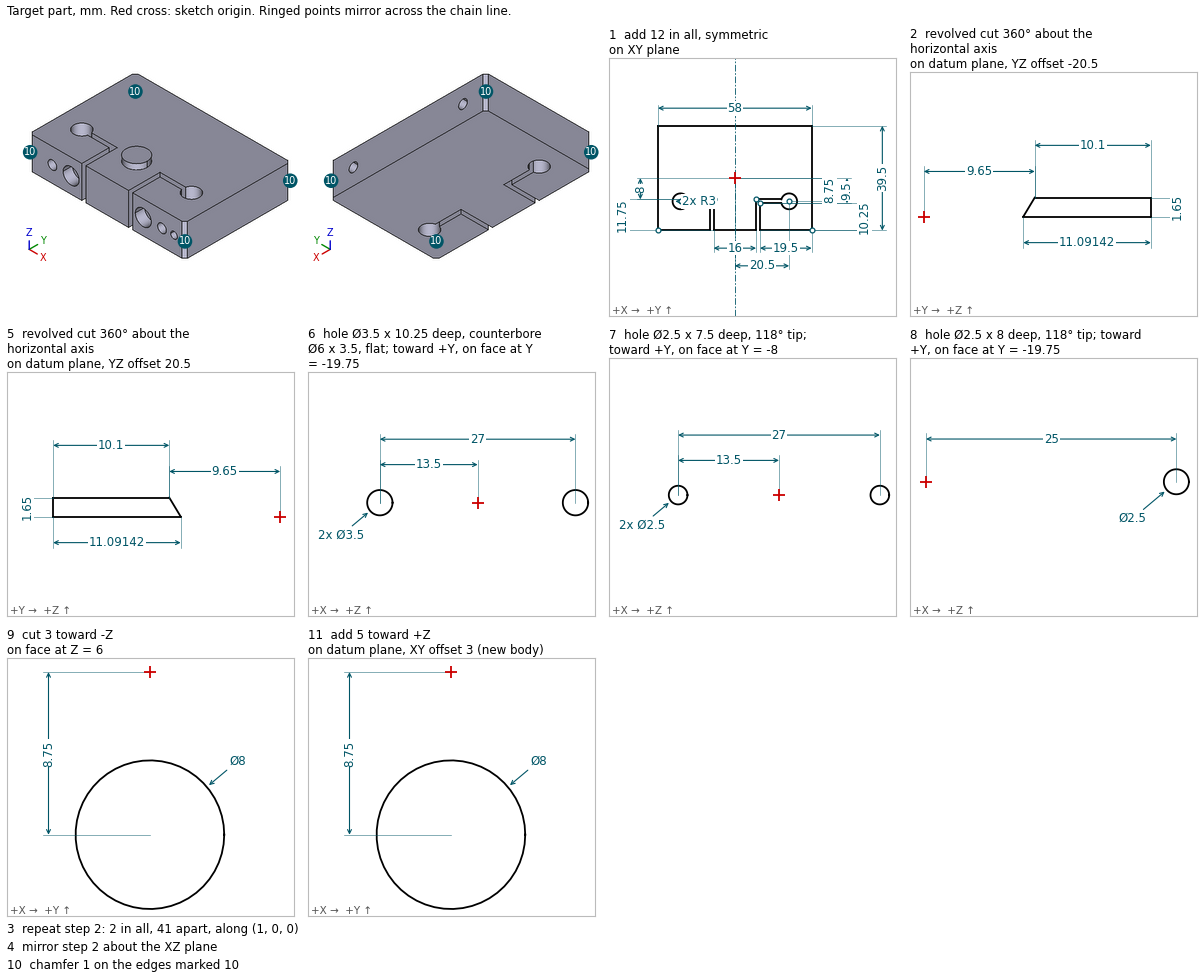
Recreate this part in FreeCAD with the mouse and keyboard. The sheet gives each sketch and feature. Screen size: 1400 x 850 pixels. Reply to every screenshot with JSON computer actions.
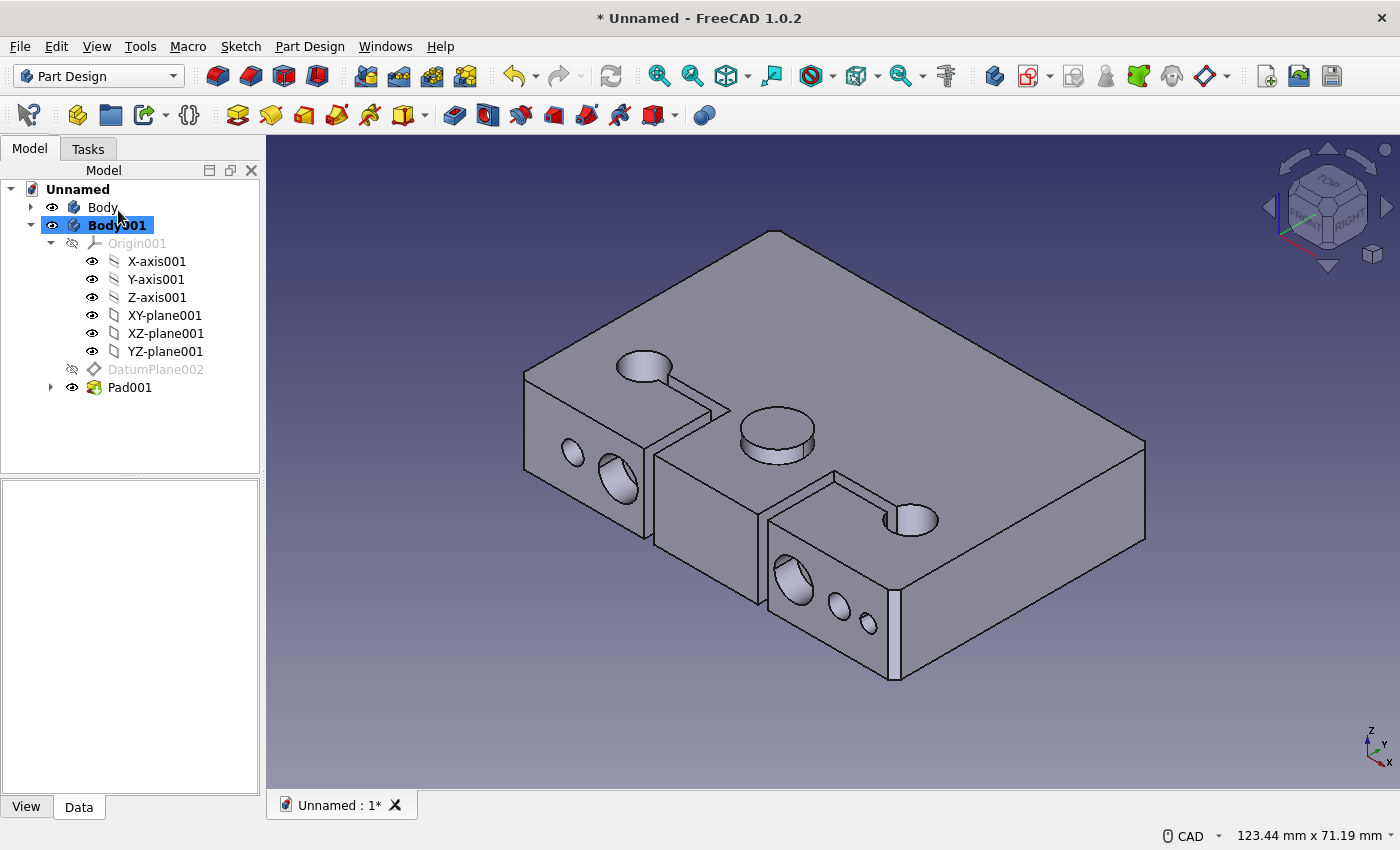
{"action": "left_click", "coordinate": [660, 76]}